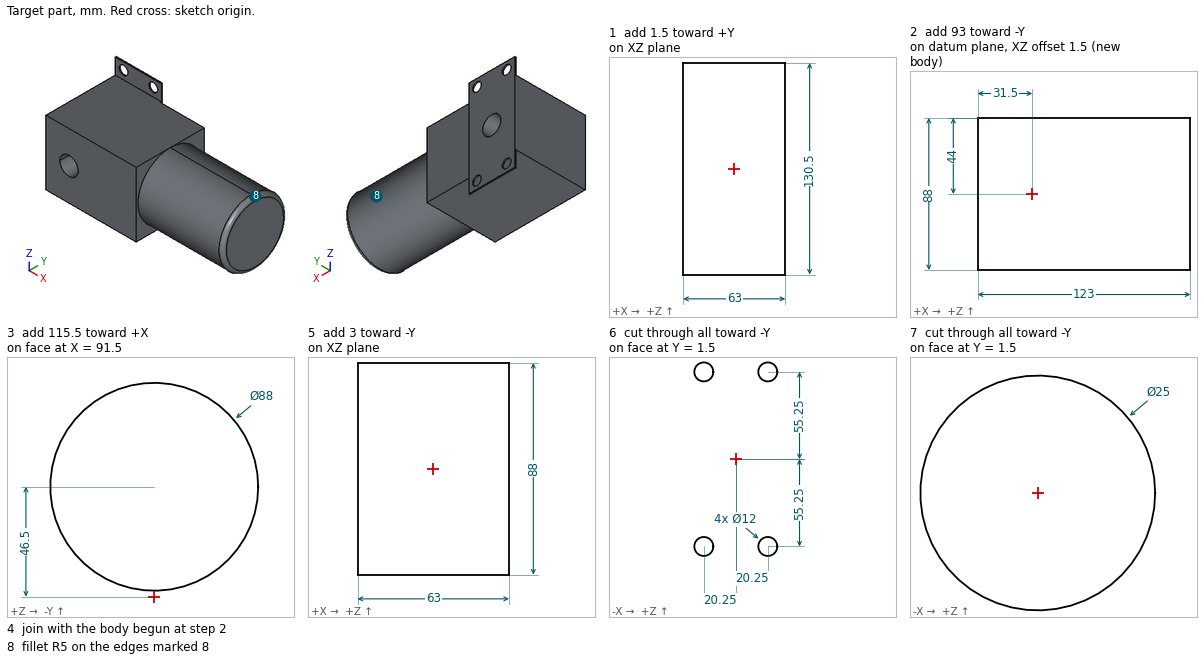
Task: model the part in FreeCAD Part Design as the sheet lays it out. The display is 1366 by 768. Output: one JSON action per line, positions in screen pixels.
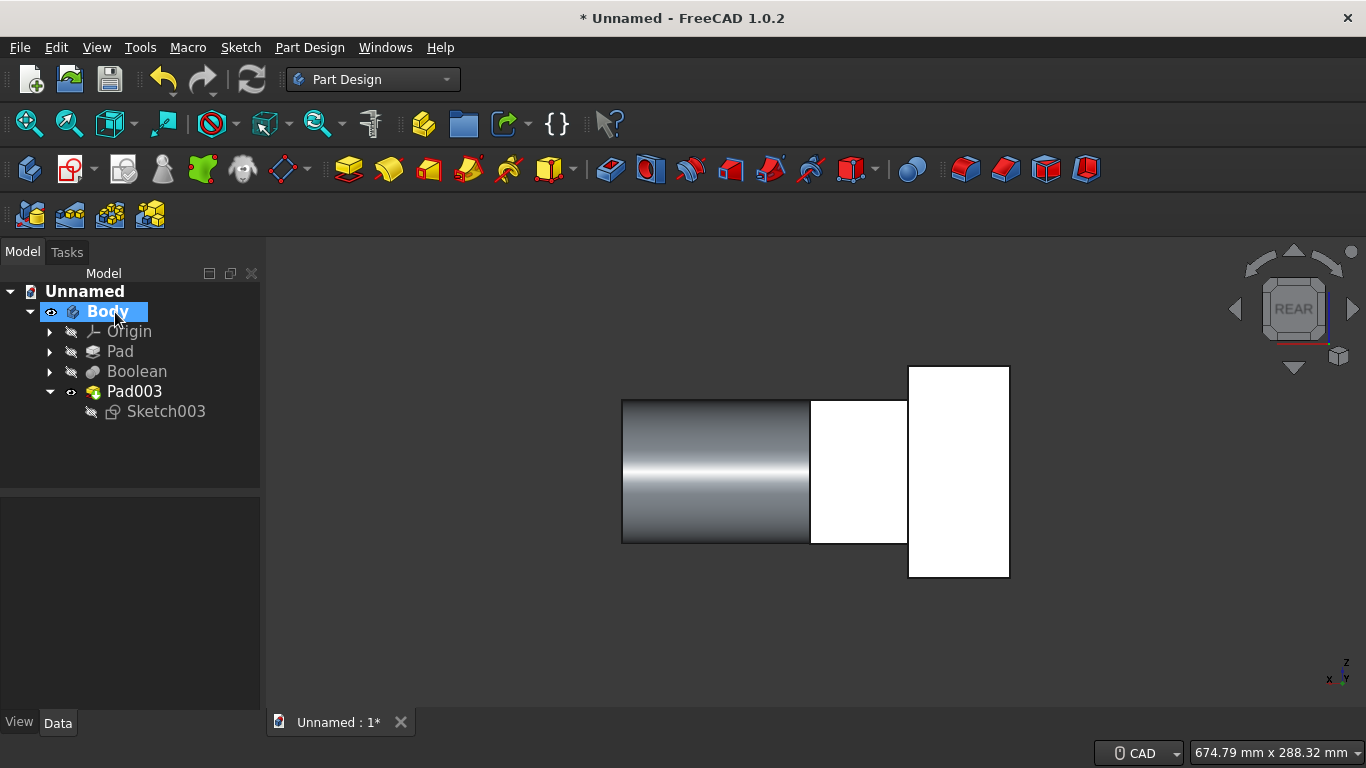
{"action": "left_click", "coordinate": [959, 441]}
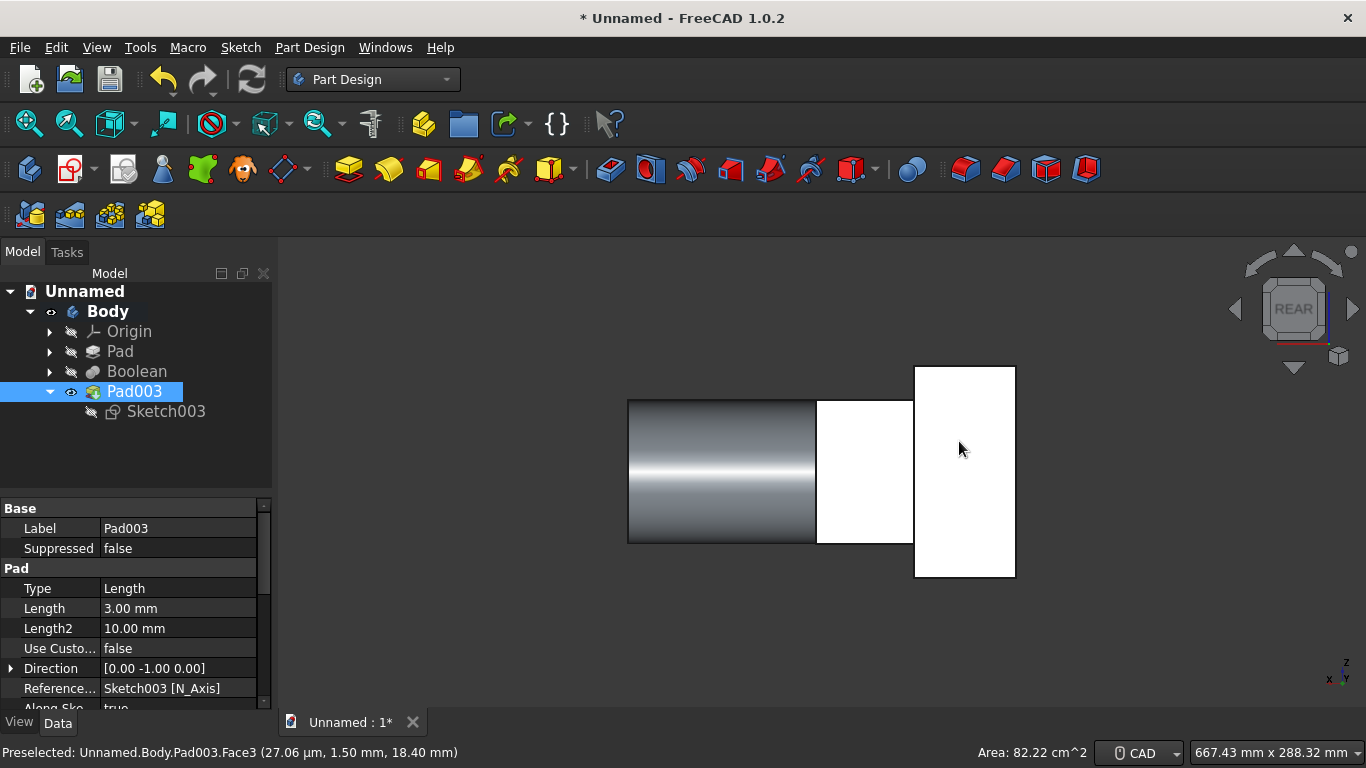
{"action": "left_click", "coordinate": [70, 170]}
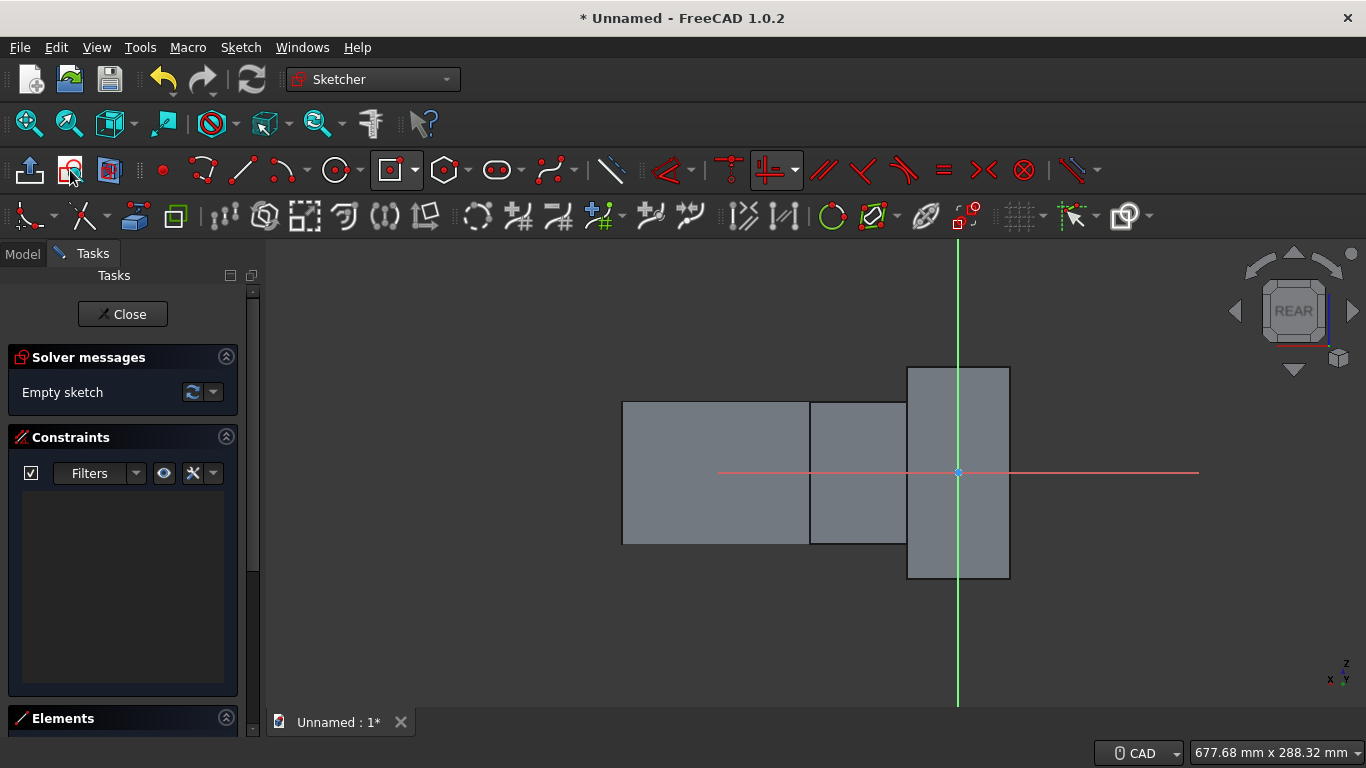
{"action": "scroll", "coordinate": [1201, 473], "scroll_direction": "up", "scroll_amount": 2}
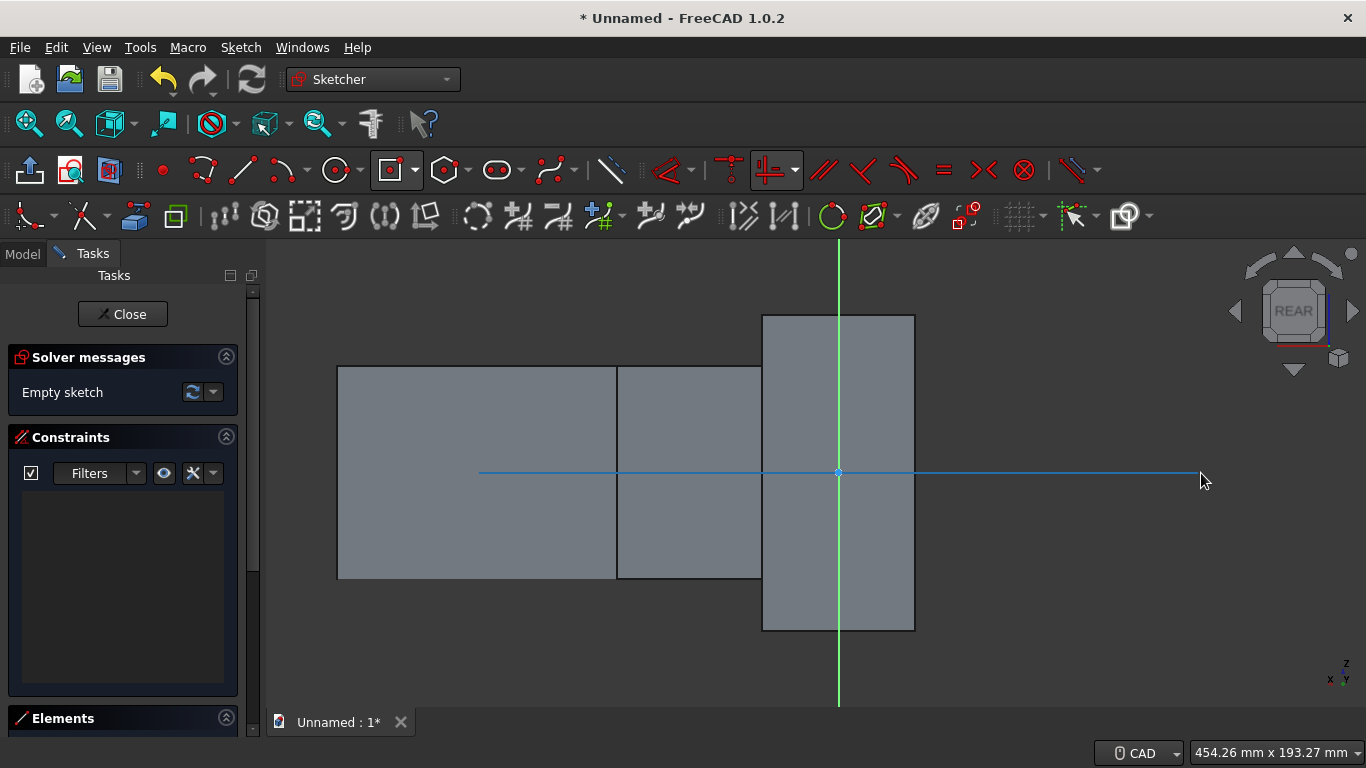
{"action": "left_click", "coordinate": [336, 170]}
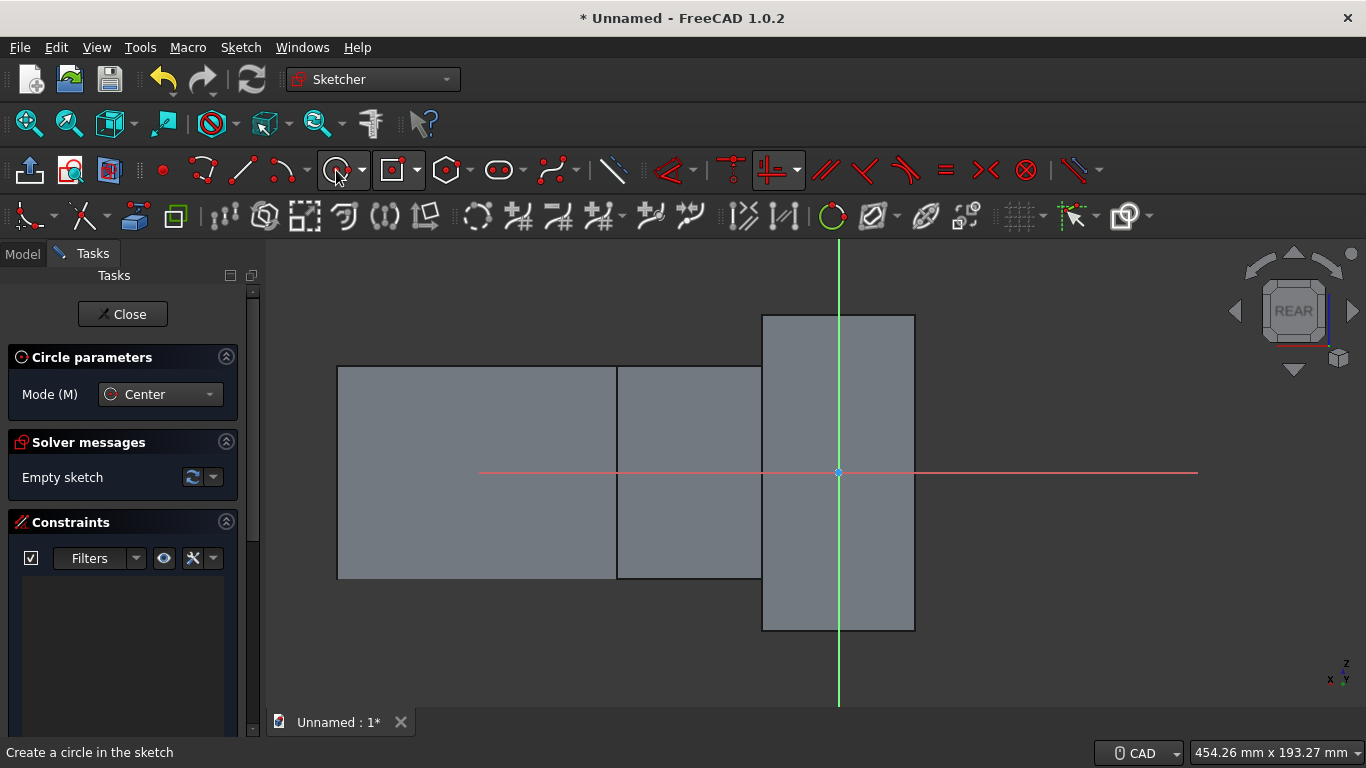
{"action": "scroll", "coordinate": [888, 607], "scroll_direction": "up", "scroll_amount": 3}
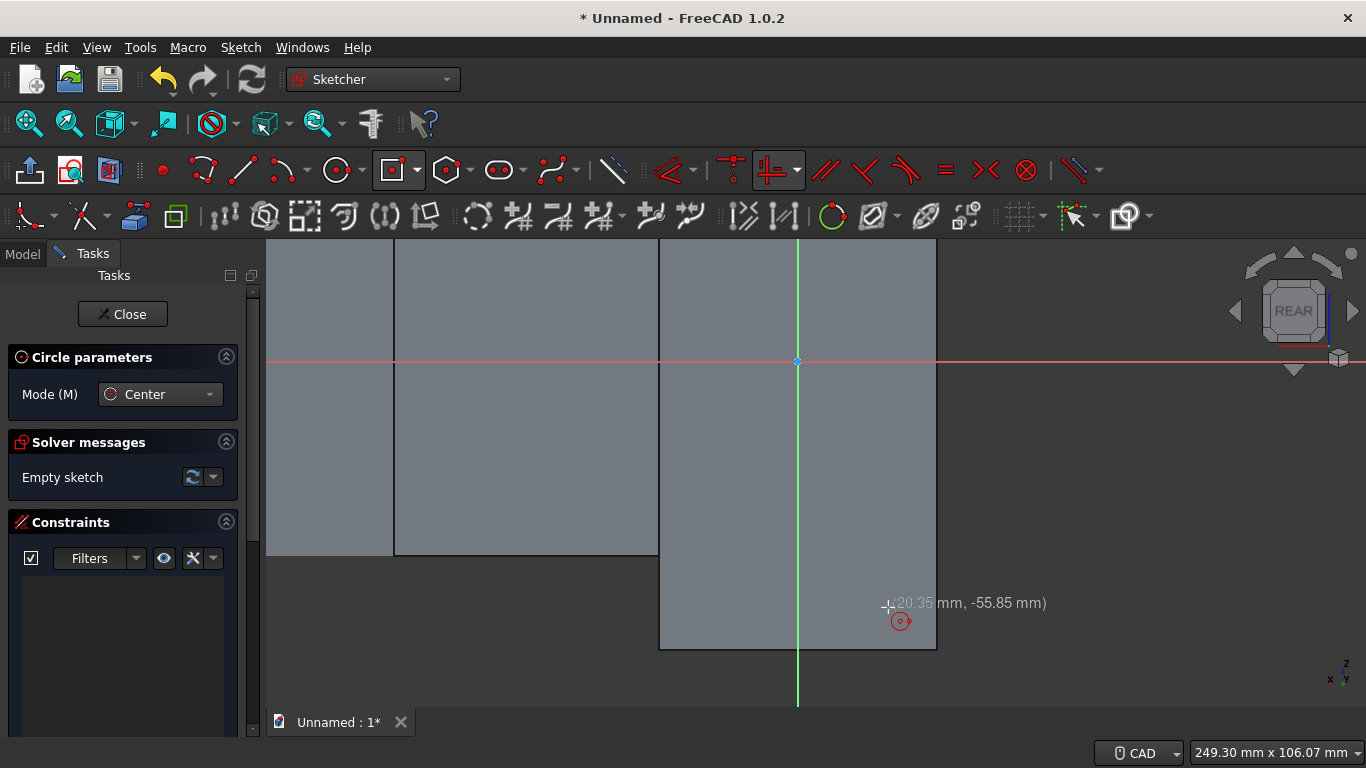
{"action": "left_click", "coordinate": [887, 606]}
{"action": "left_click", "coordinate": [906, 587]}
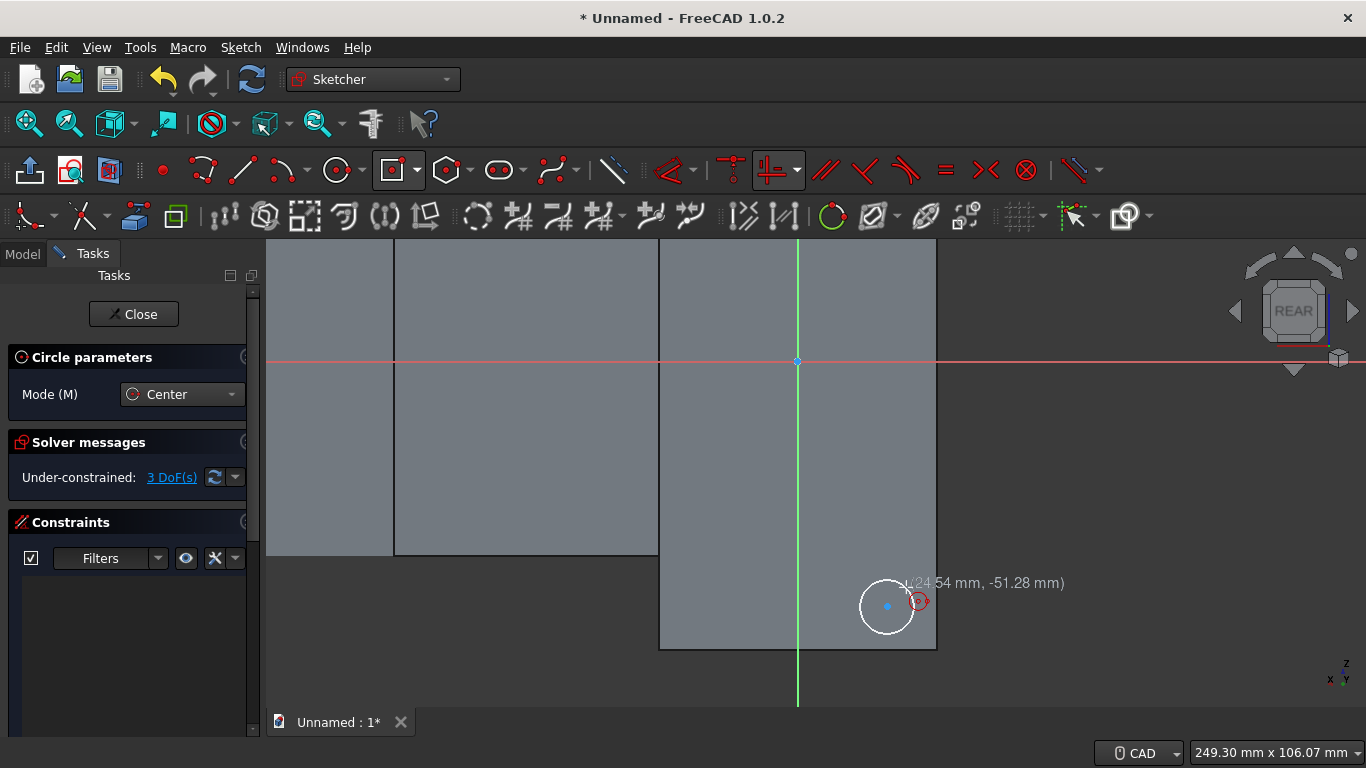
{"action": "left_click", "coordinate": [708, 606]}
{"action": "left_click", "coordinate": [727, 587]}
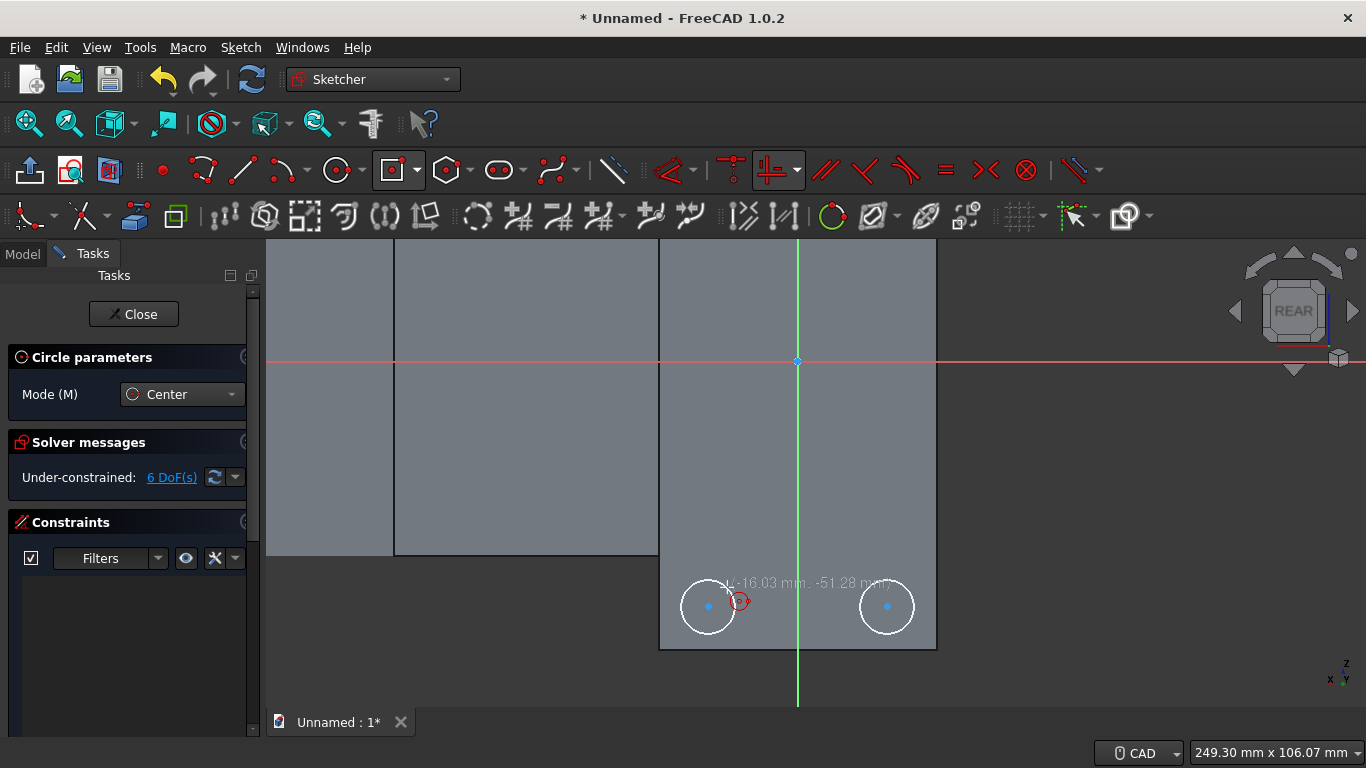
{"action": "scroll", "coordinate": [686, 608], "scroll_direction": "down", "scroll_amount": 3}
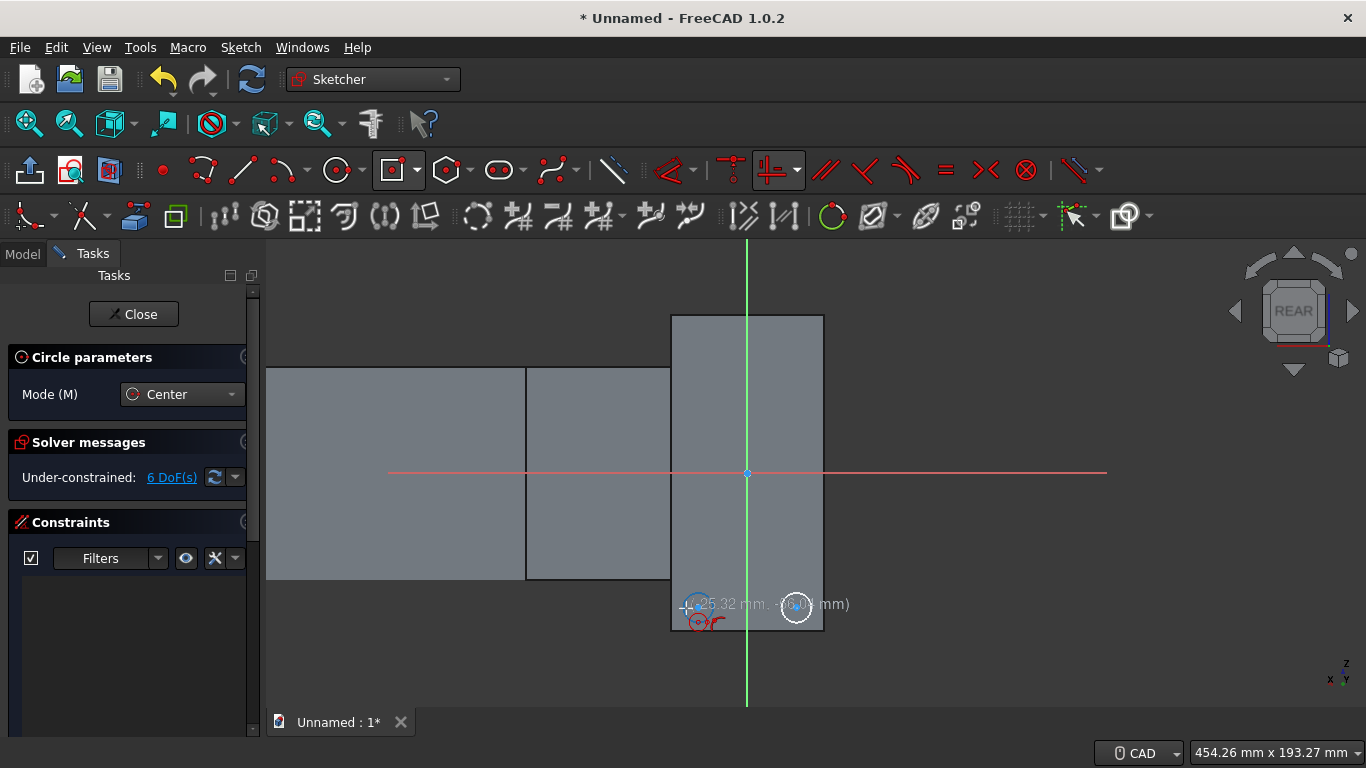
{"action": "scroll", "coordinate": [797, 339], "scroll_direction": "up", "scroll_amount": 3}